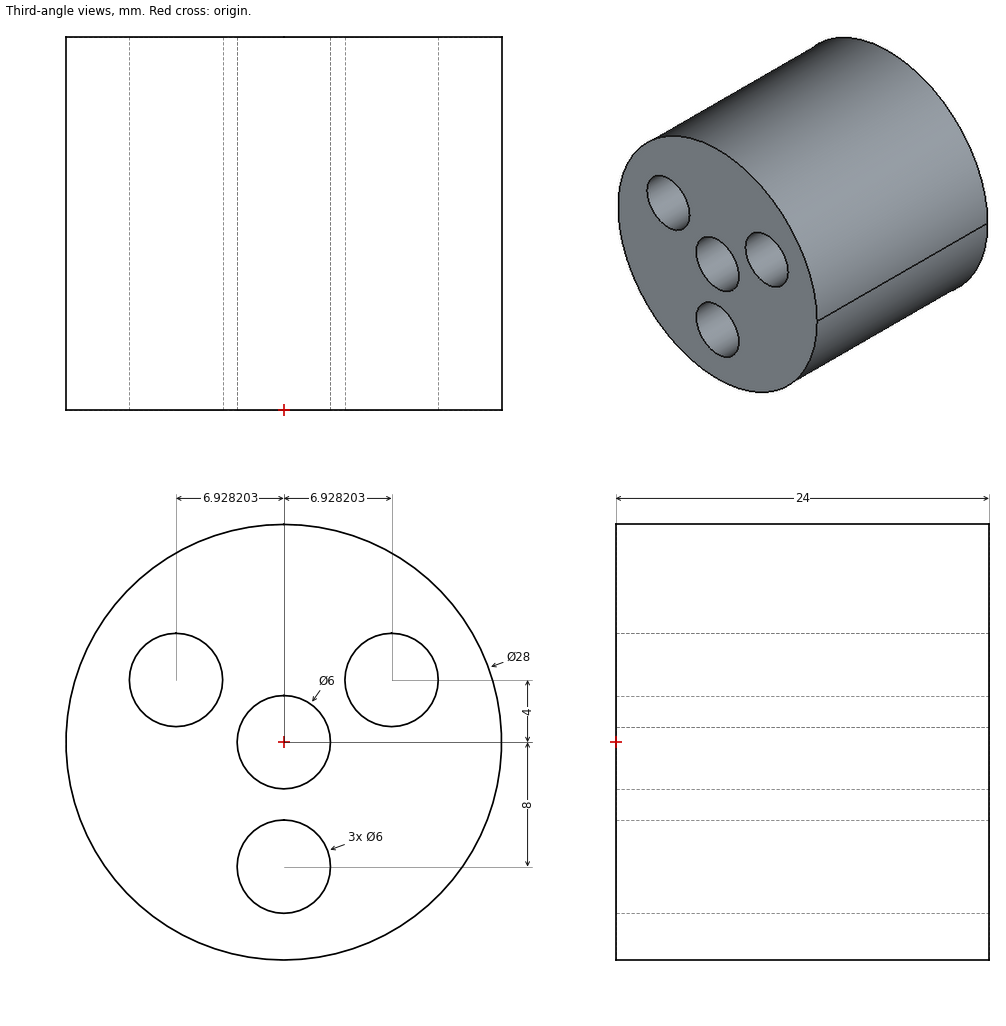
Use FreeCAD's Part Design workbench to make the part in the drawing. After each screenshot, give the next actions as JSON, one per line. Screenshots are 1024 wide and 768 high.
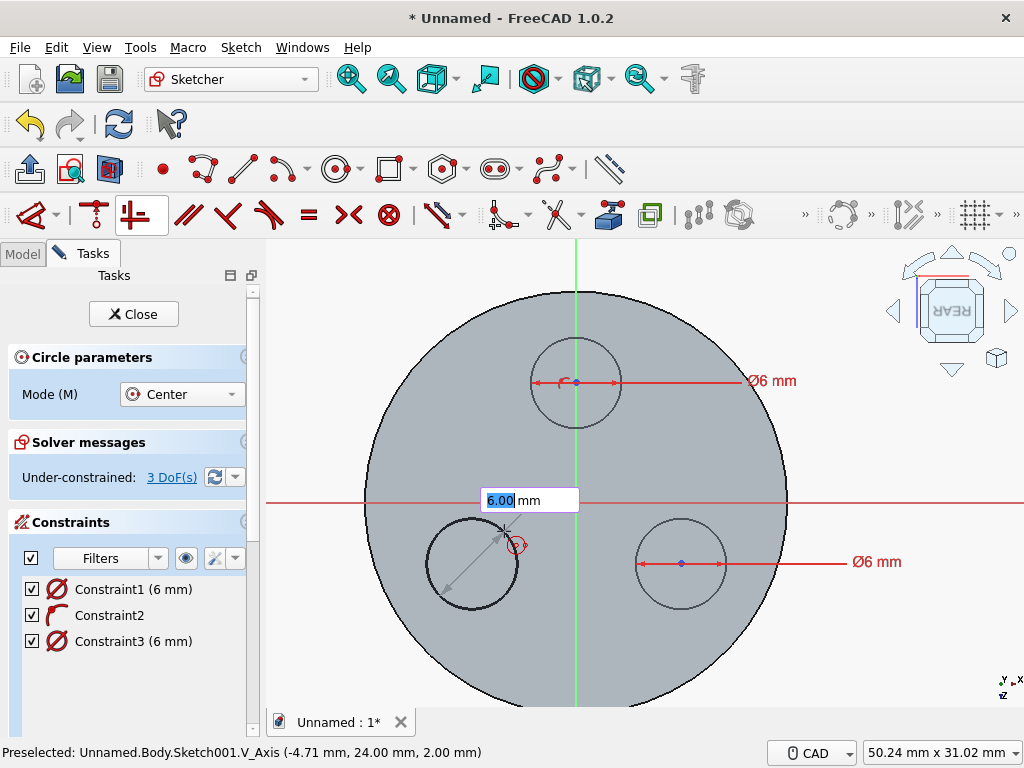
{"action": "type", "text": "6"}
{"action": "key", "text": "Return"}
{"action": "key", "text": "Escape"}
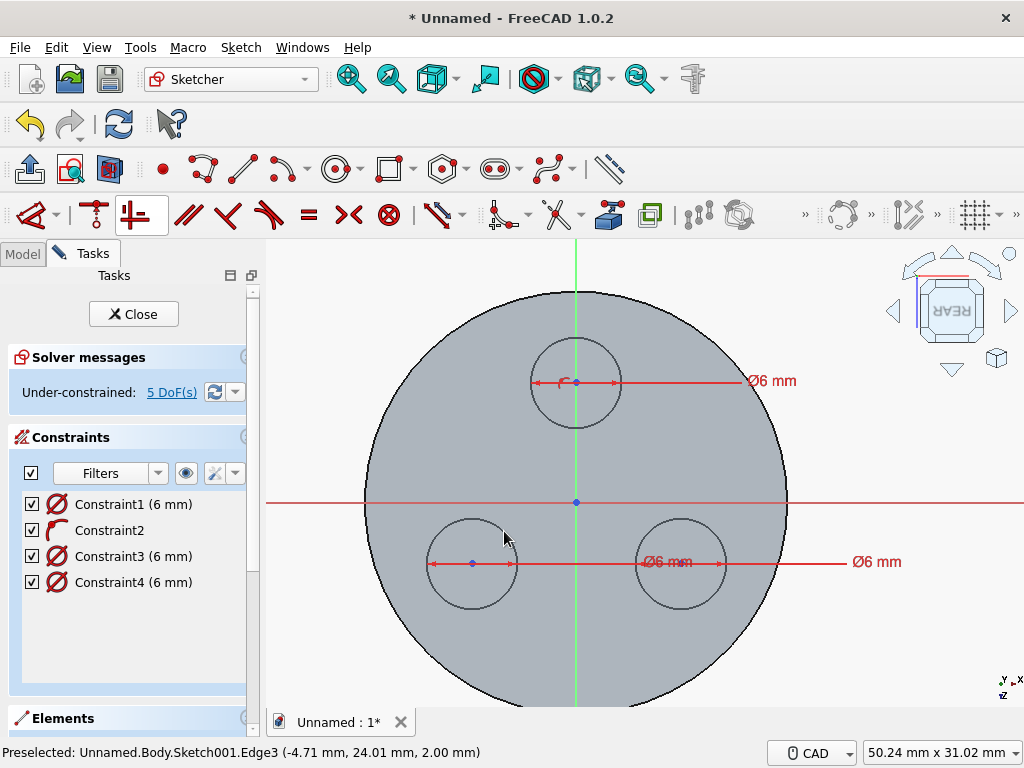
{"action": "left_click", "coordinate": [681, 564]}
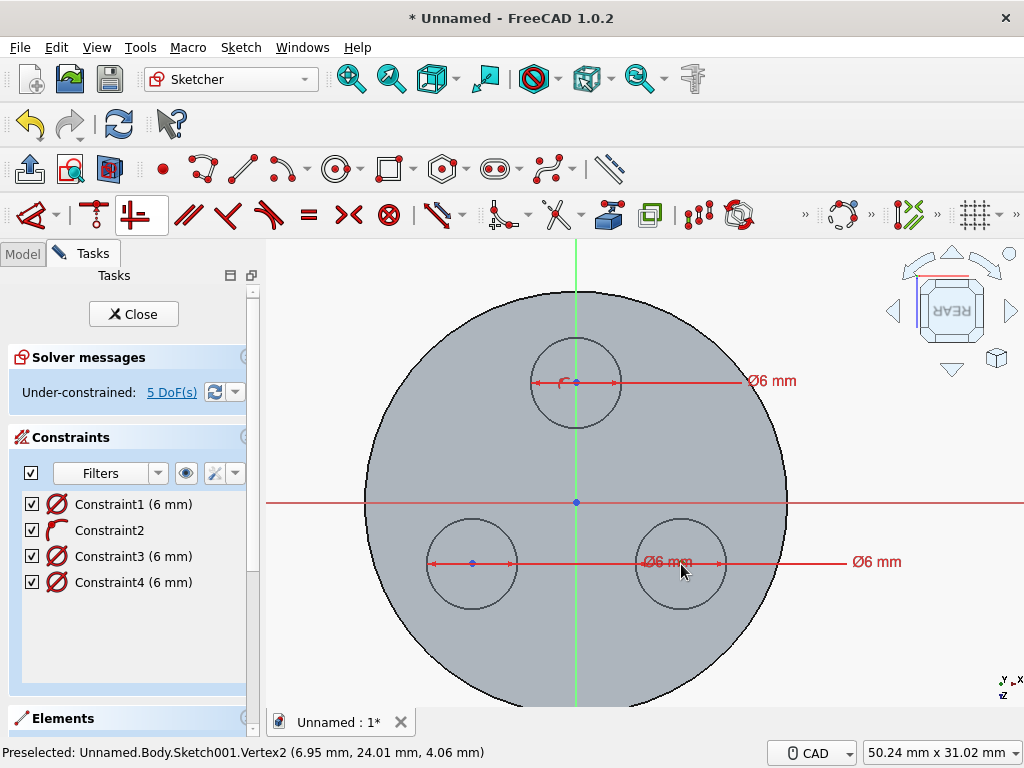
{"action": "left_click", "coordinate": [472, 564]}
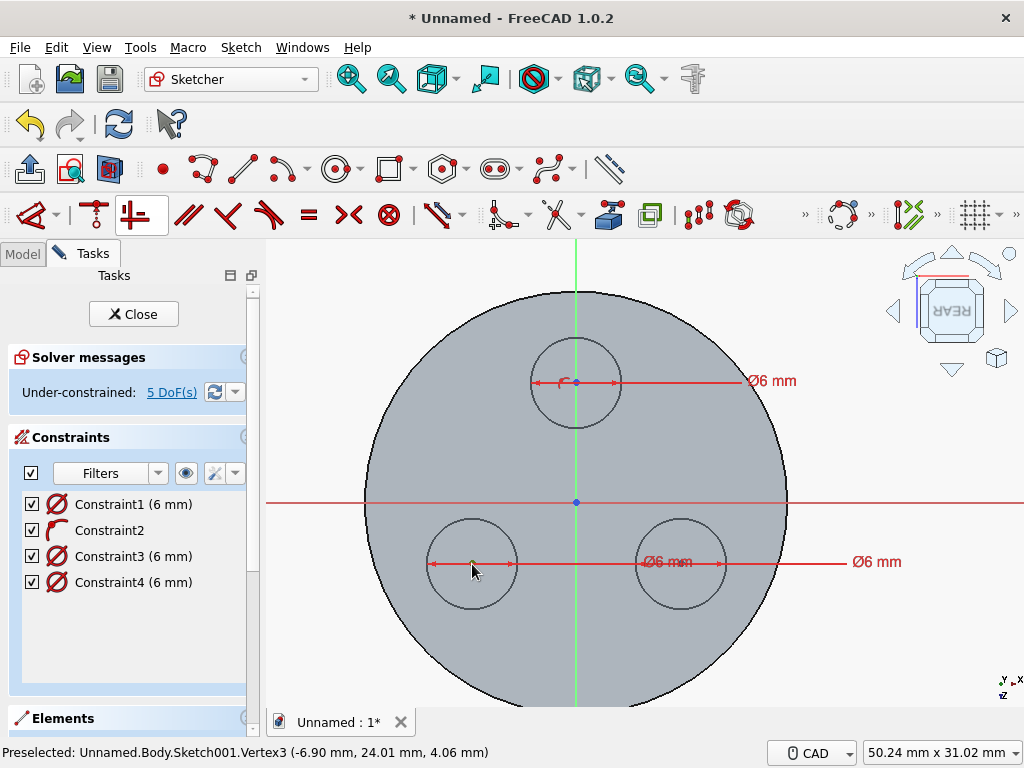
{"action": "key", "text": "h"}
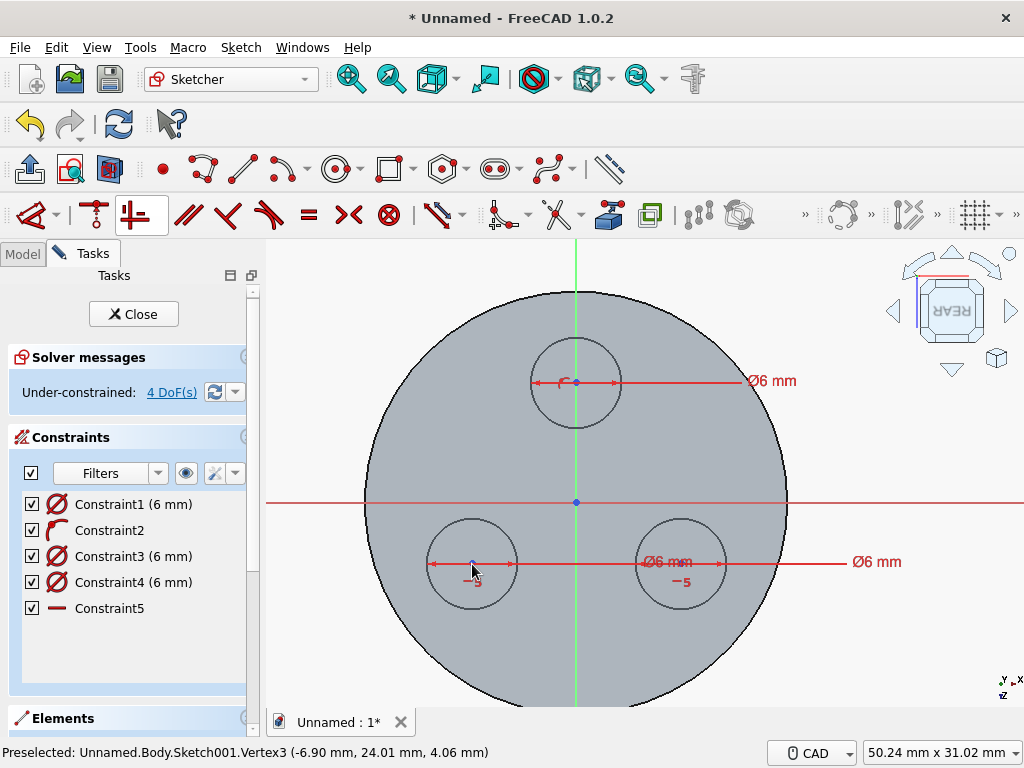
{"action": "key", "text": "d"}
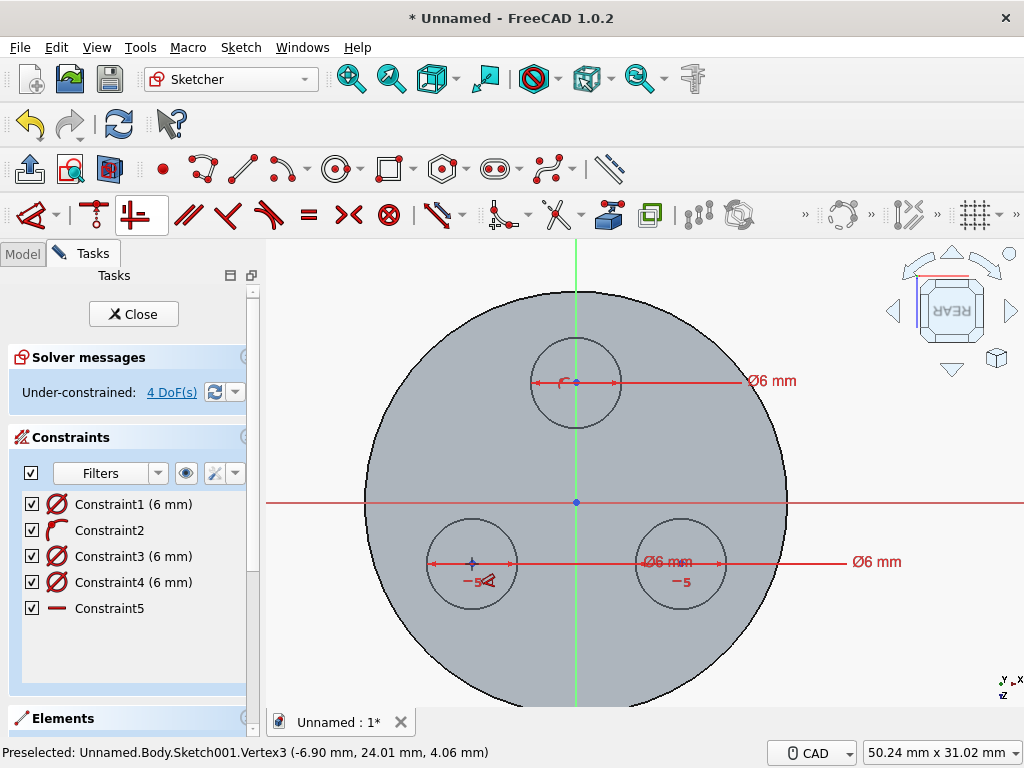
{"action": "left_click", "coordinate": [576, 383]}
{"action": "left_click", "coordinate": [610, 443]}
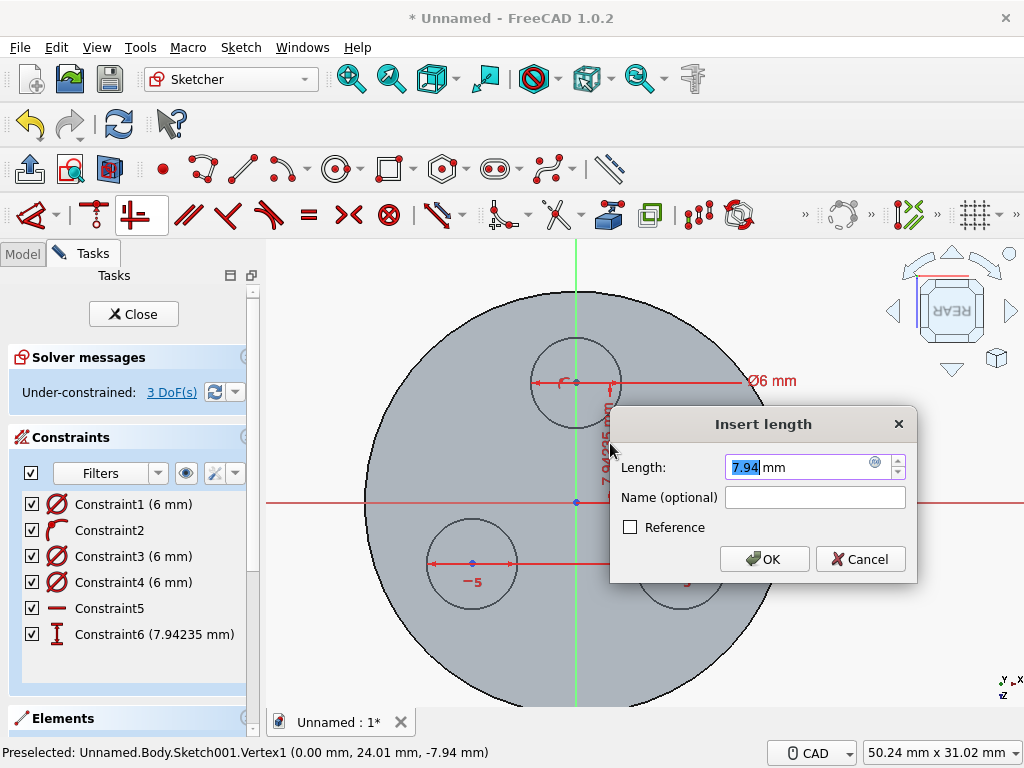
{"action": "type", "text": "8"}
{"action": "key", "text": "Return"}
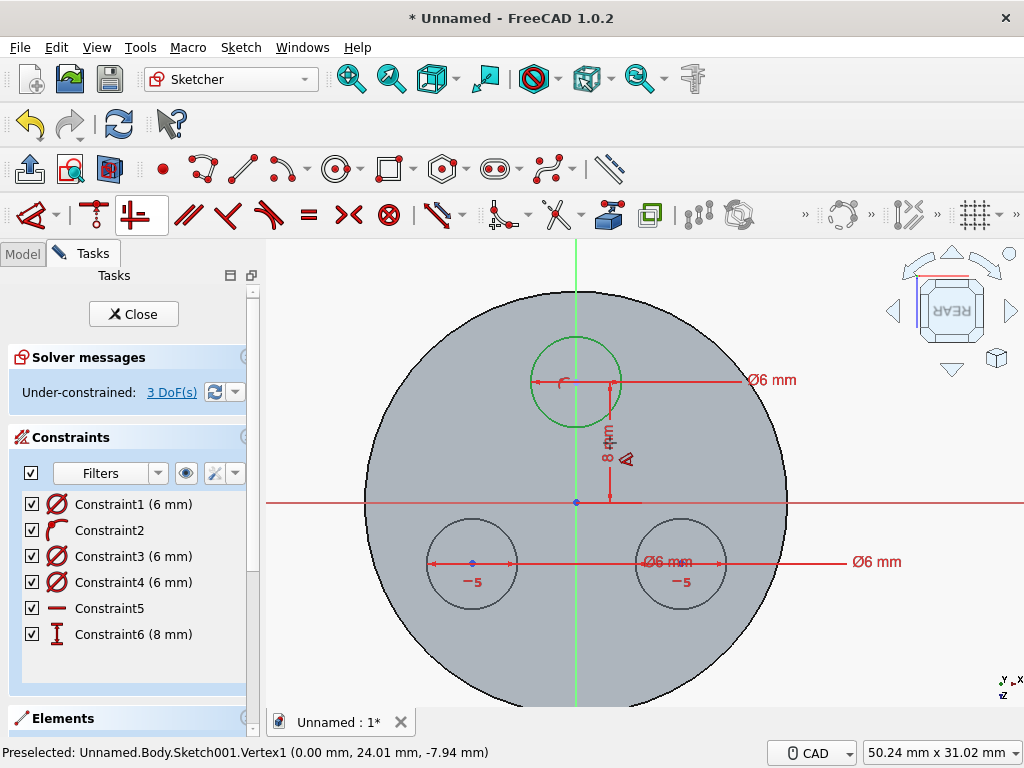
{"action": "left_click", "coordinate": [681, 564]}
{"action": "left_click", "coordinate": [542, 533]}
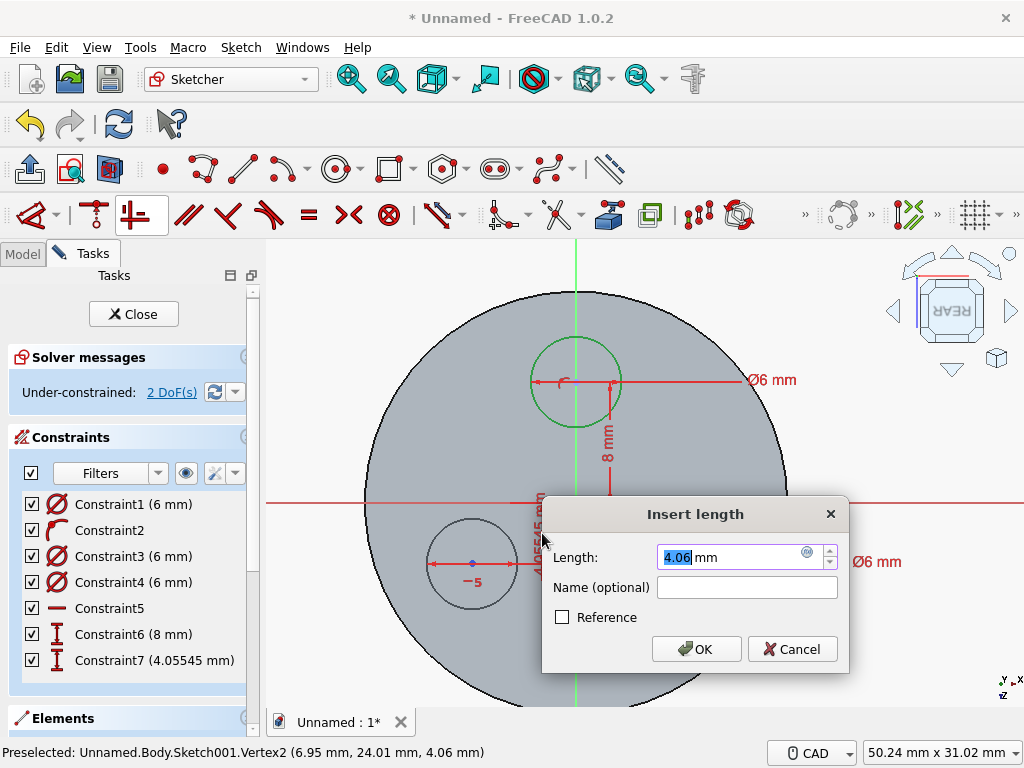
{"action": "type", "text": "4"}
{"action": "key", "text": "Return"}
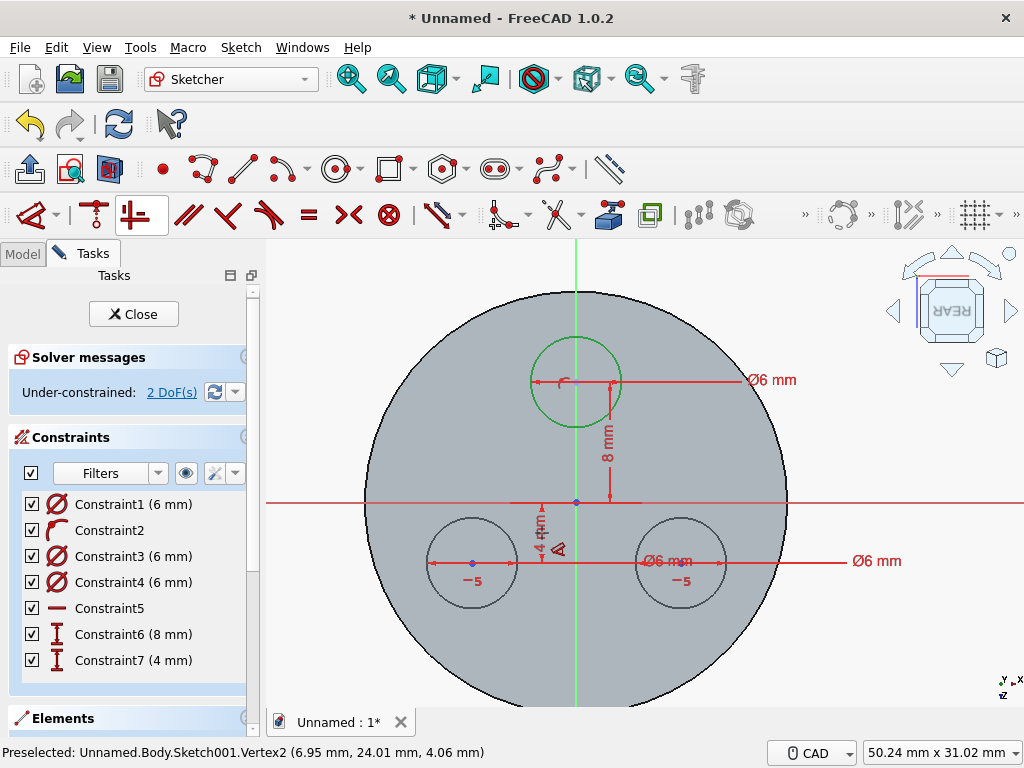
{"action": "left_click", "coordinate": [681, 563]}
{"action": "left_click", "coordinate": [629, 597]}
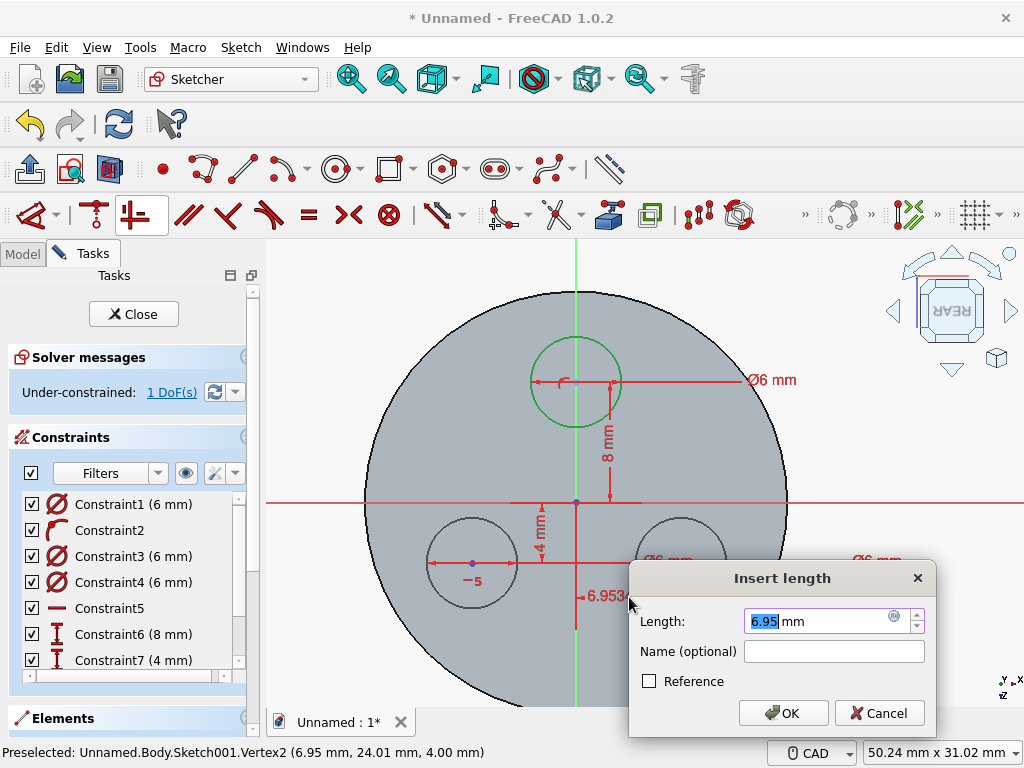
{"action": "type", "text": "6.928203"}
{"action": "key", "text": "Return"}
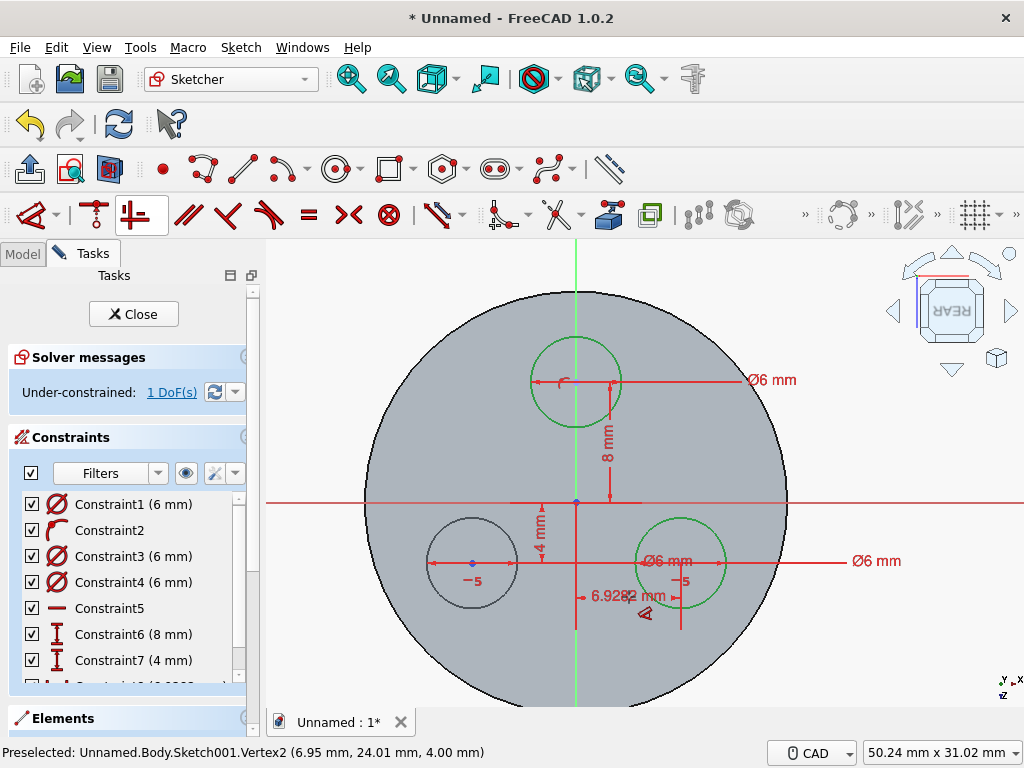
{"action": "left_click", "coordinate": [472, 563]}
{"action": "left_click", "coordinate": [524, 597]}